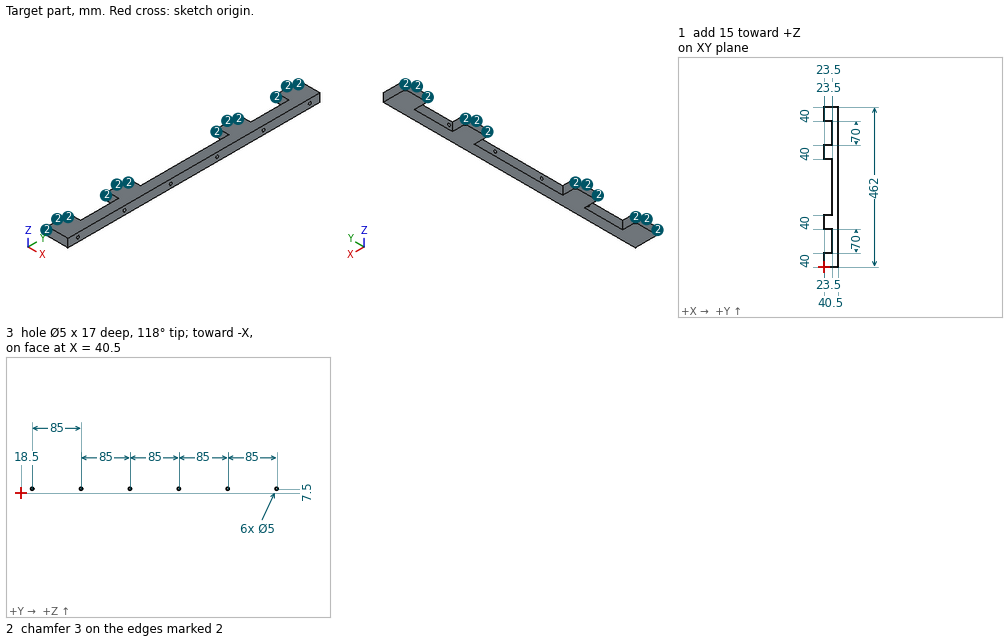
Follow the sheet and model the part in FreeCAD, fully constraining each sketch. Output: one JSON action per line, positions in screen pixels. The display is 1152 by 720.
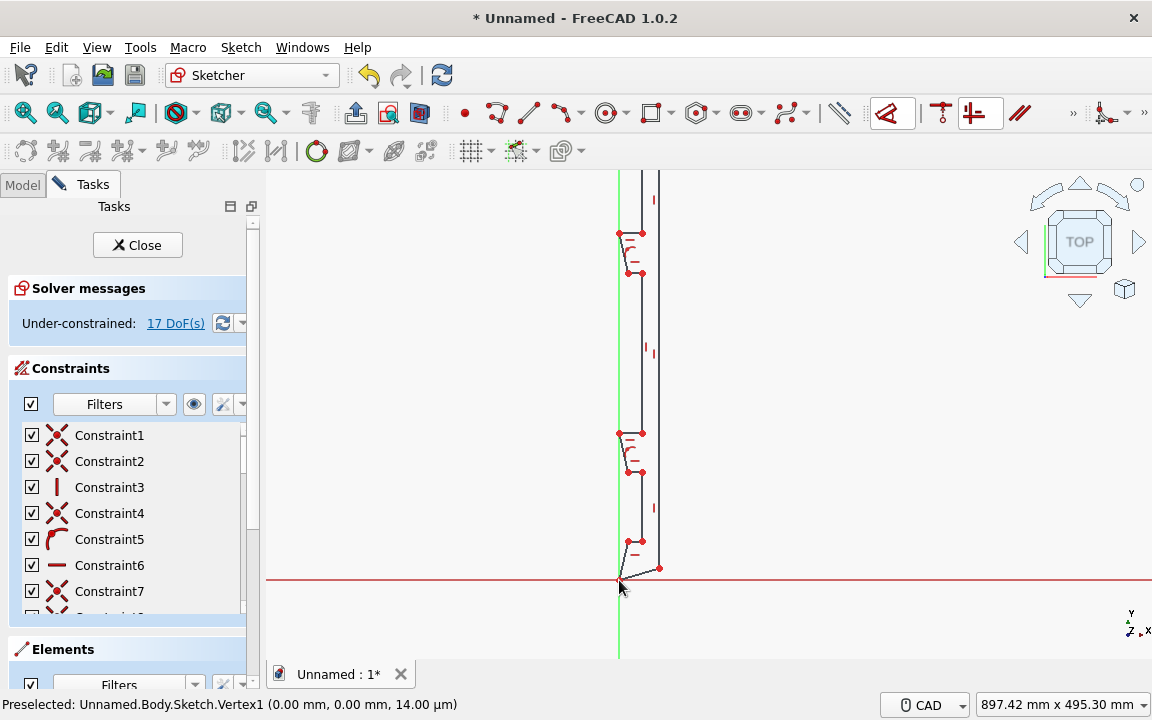
{"action": "scroll", "coordinate": [631, 577], "scroll_direction": "up", "scroll_amount": 2}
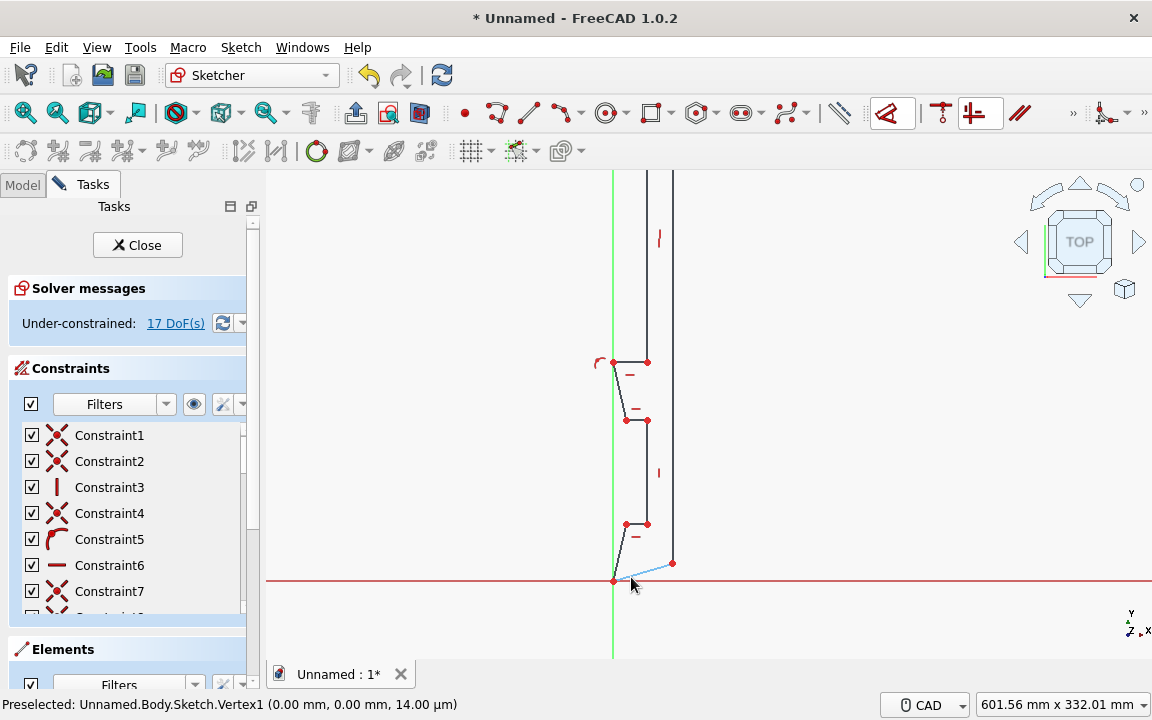
{"action": "left_click", "coordinate": [631, 576]}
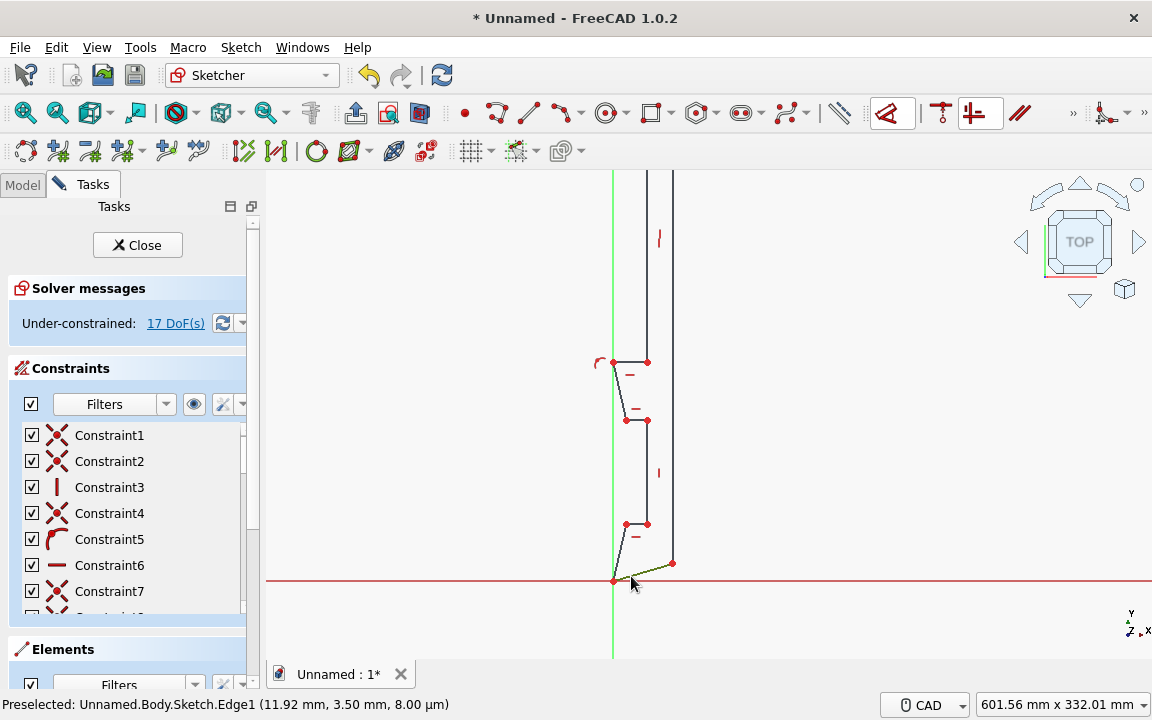
{"action": "left_click", "coordinate": [998, 114]}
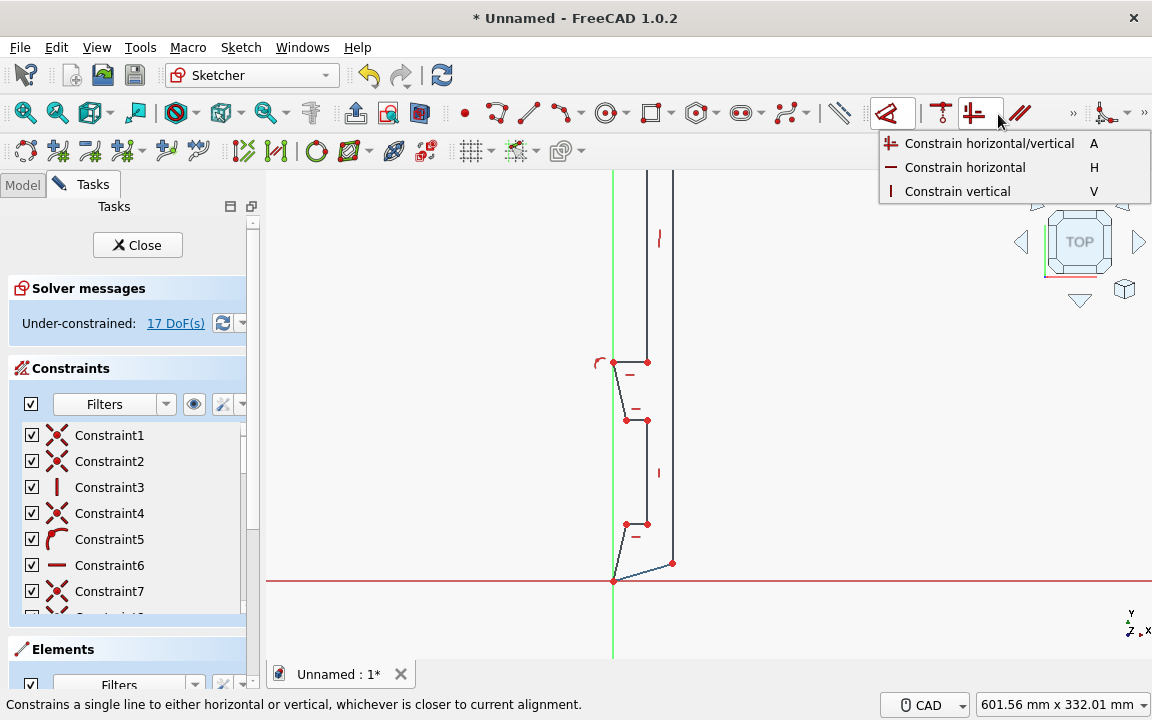
{"action": "left_click", "coordinate": [1015, 167]}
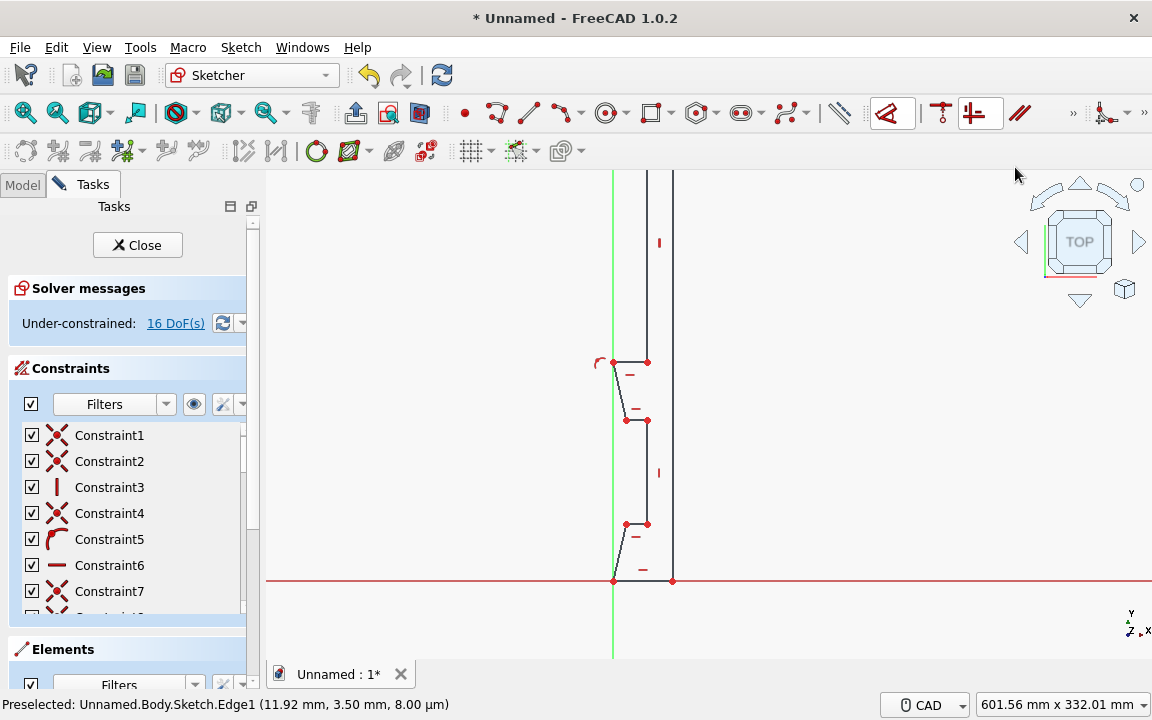
{"action": "scroll", "coordinate": [638, 556], "scroll_direction": "down", "scroll_amount": 4}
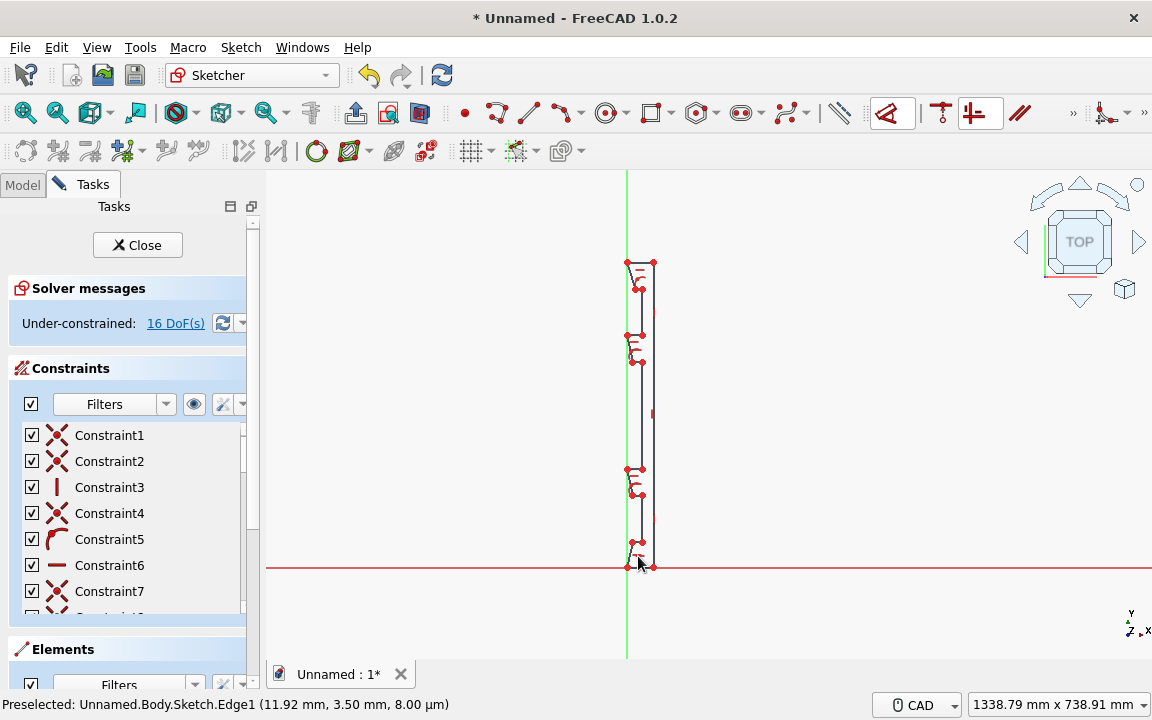
{"action": "scroll", "coordinate": [633, 282], "scroll_direction": "up", "scroll_amount": 5}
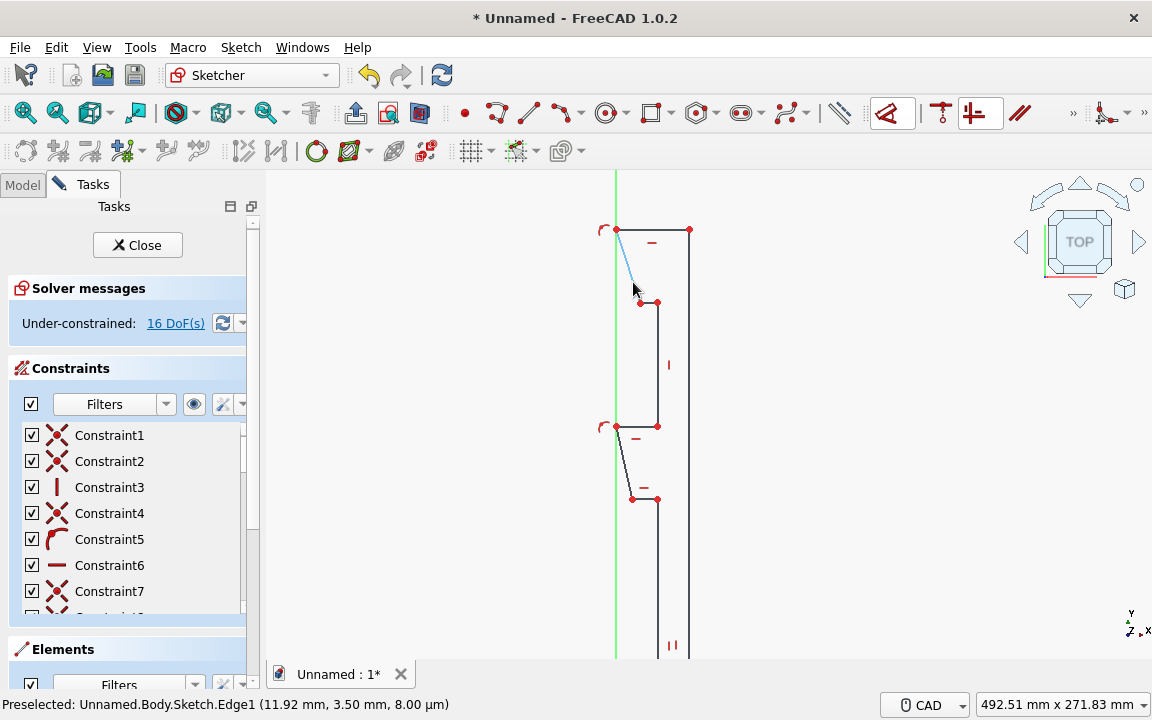
{"action": "left_click", "coordinate": [633, 281]}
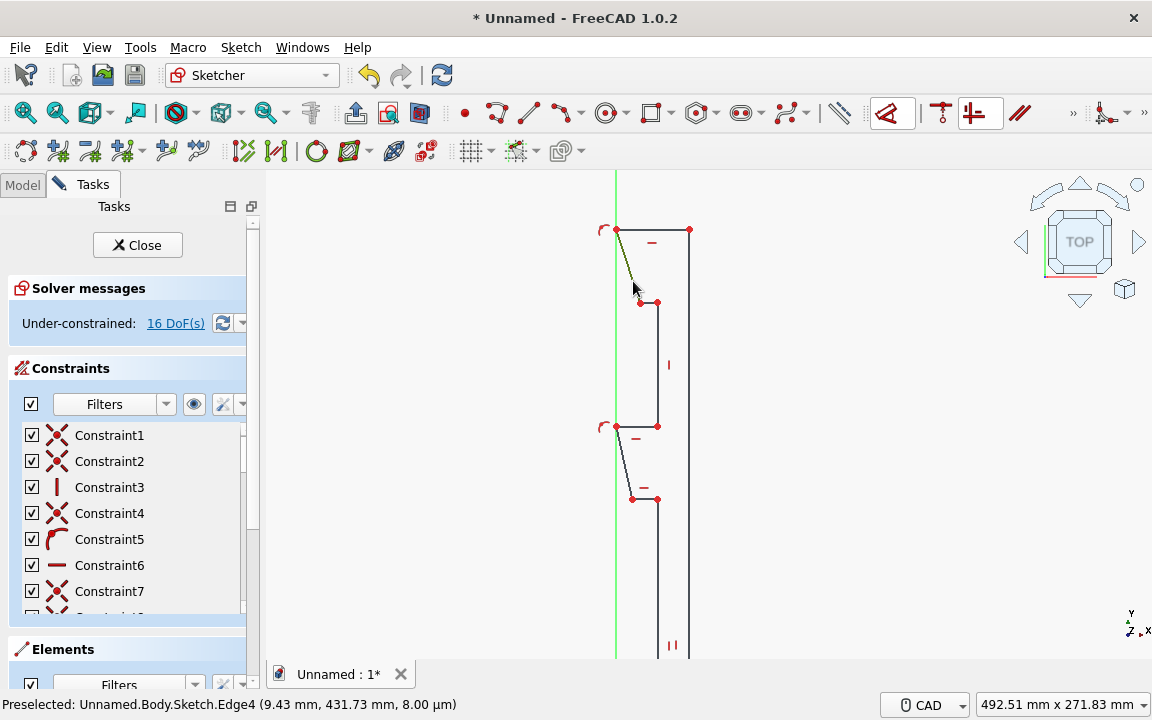
{"action": "key", "text": "v"}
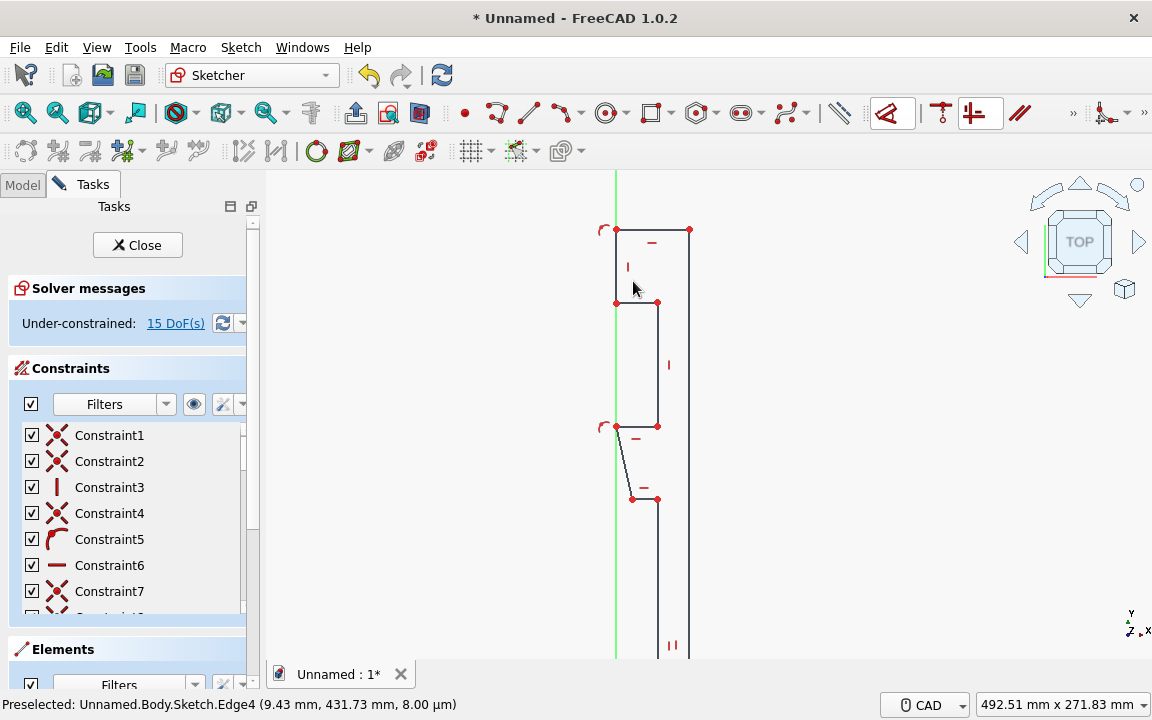
{"action": "left_click", "coordinate": [629, 303]}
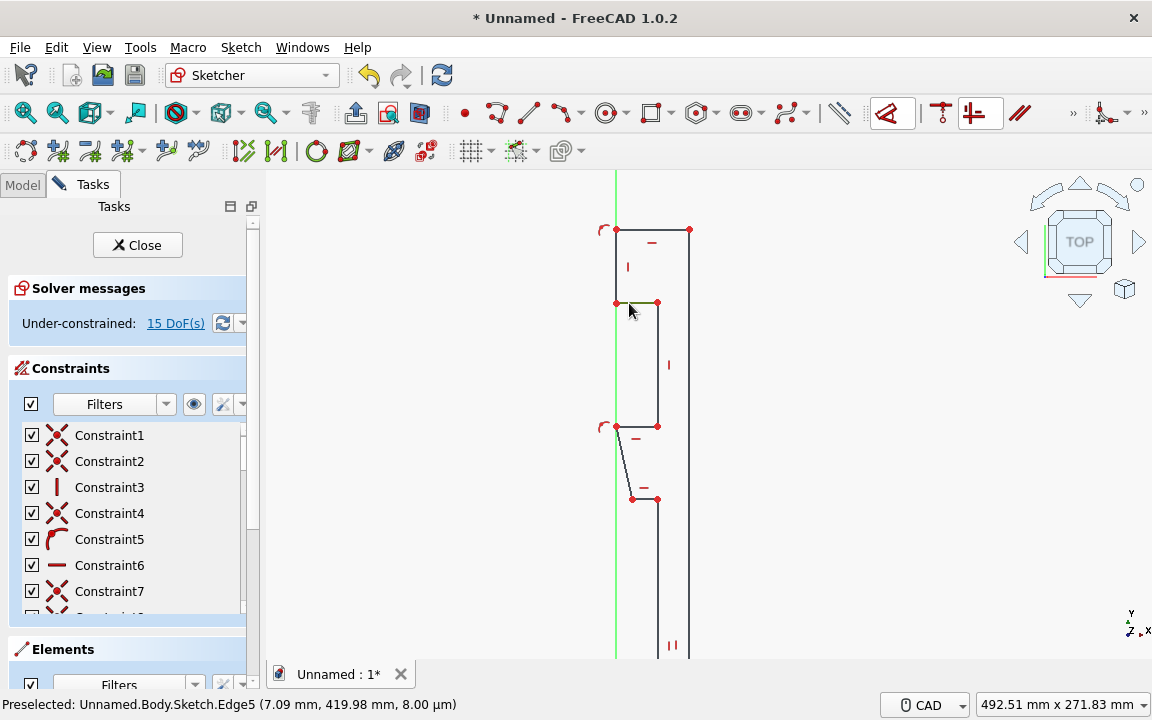
{"action": "left_click", "coordinate": [998, 114]}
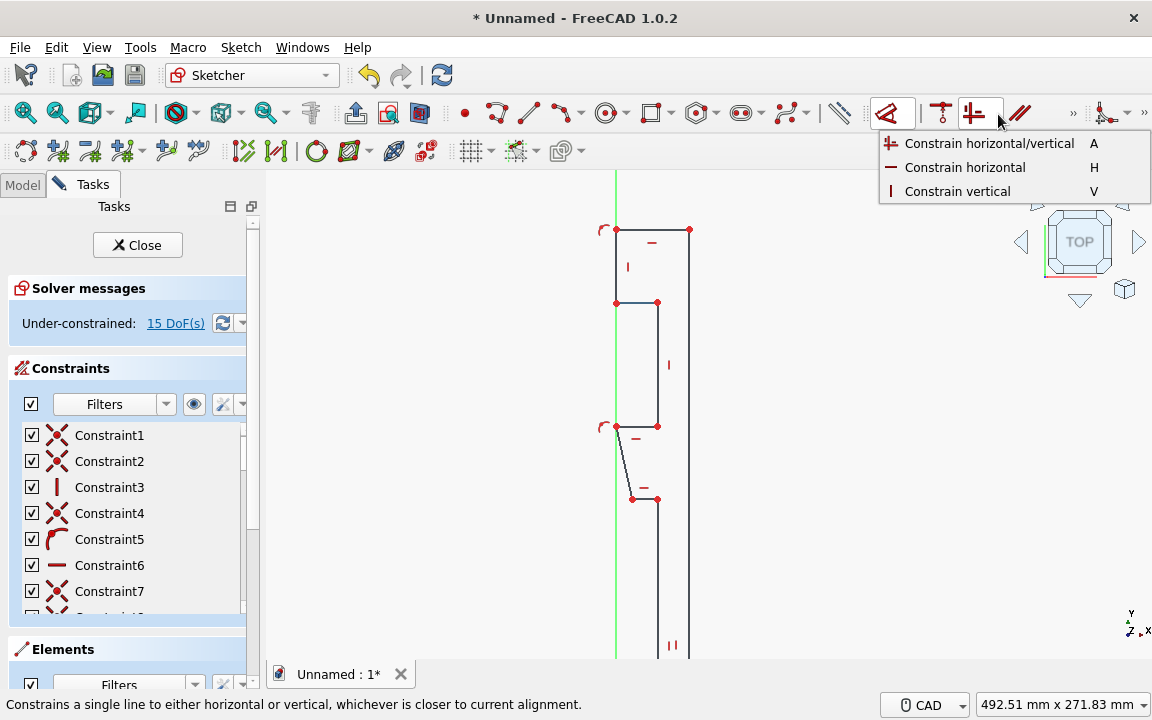
{"action": "left_click", "coordinate": [1015, 167]}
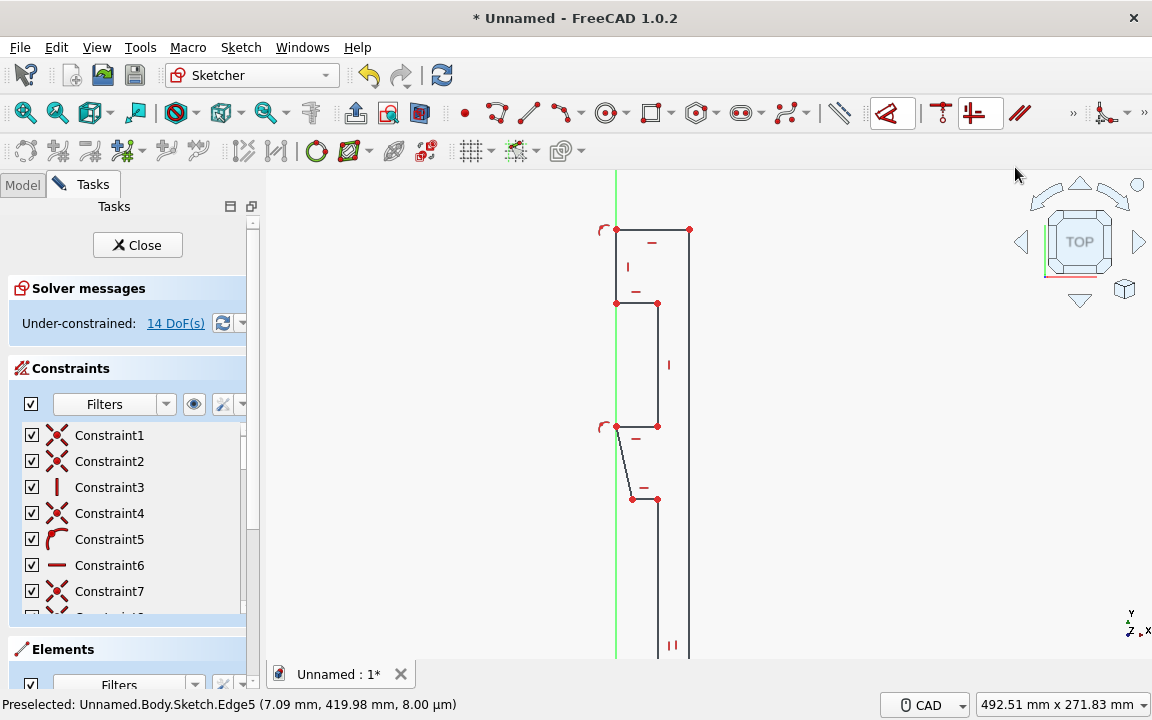
{"action": "scroll", "coordinate": [627, 478], "scroll_direction": "up", "scroll_amount": 2}